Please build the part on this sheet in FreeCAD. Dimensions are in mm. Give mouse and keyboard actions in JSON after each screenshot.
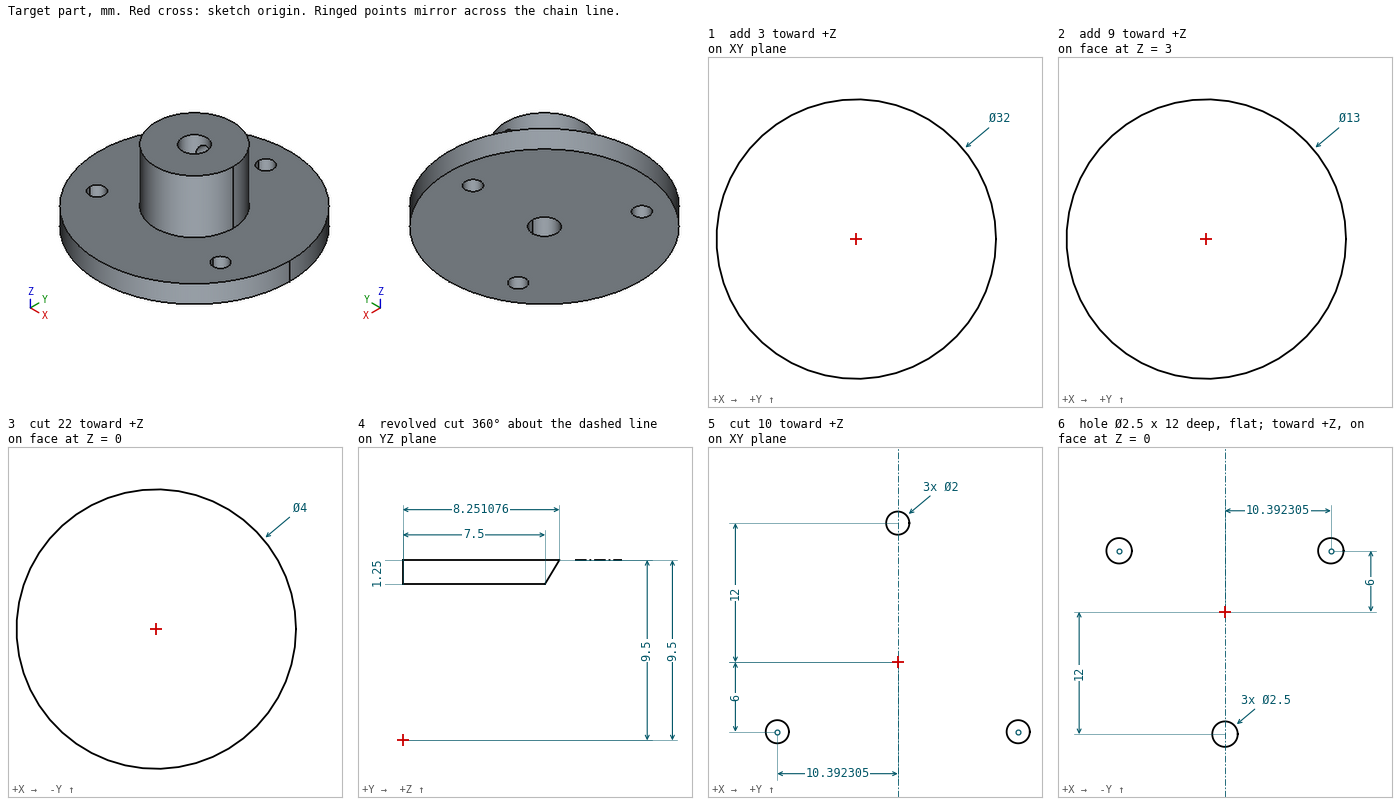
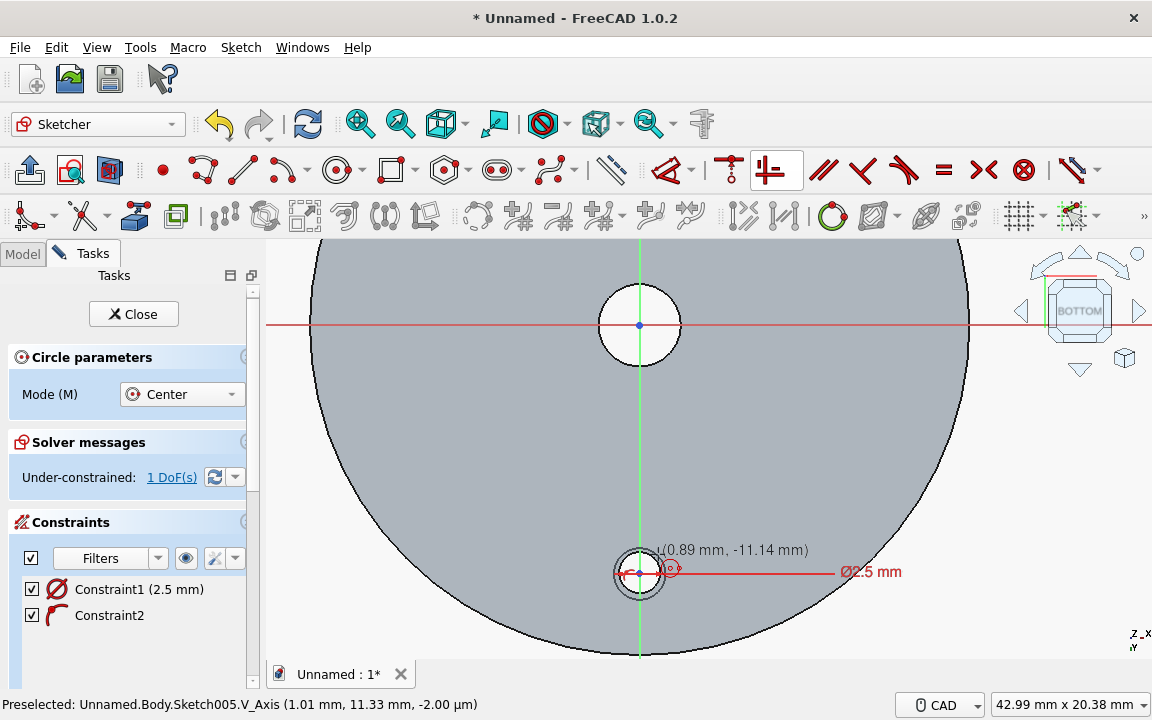
{"action": "scroll", "coordinate": [642, 575], "scroll_direction": "down", "scroll_amount": 2}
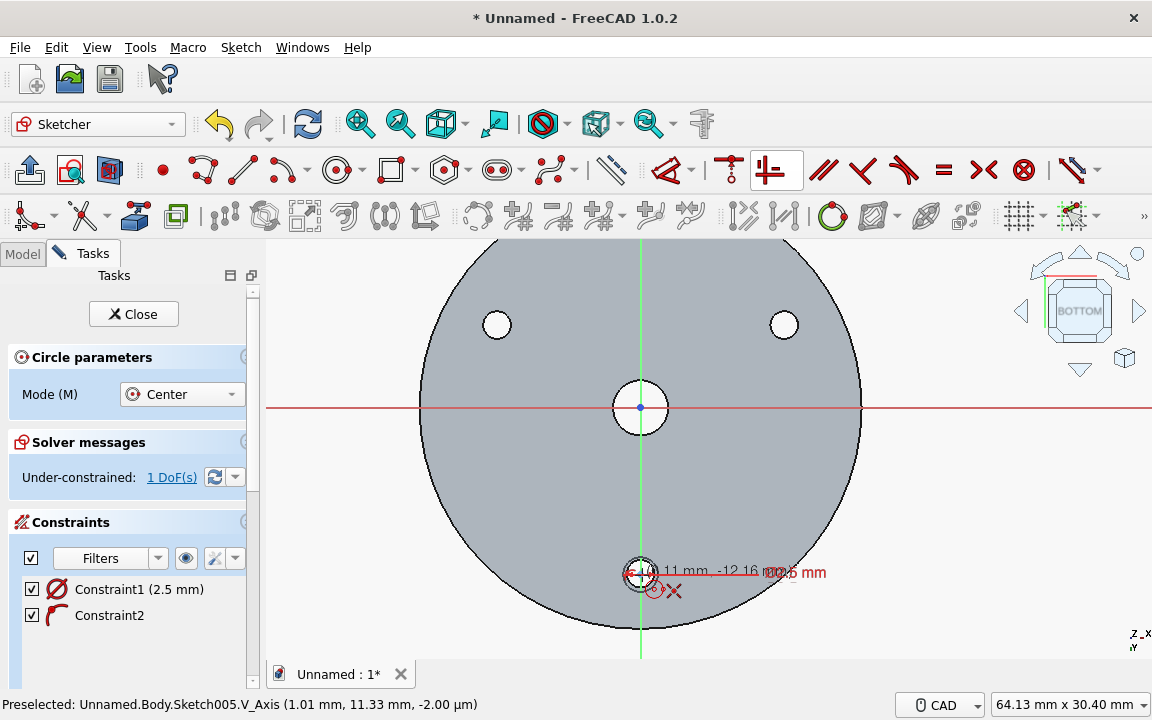
{"action": "scroll", "coordinate": [784, 325], "scroll_direction": "up", "scroll_amount": 2}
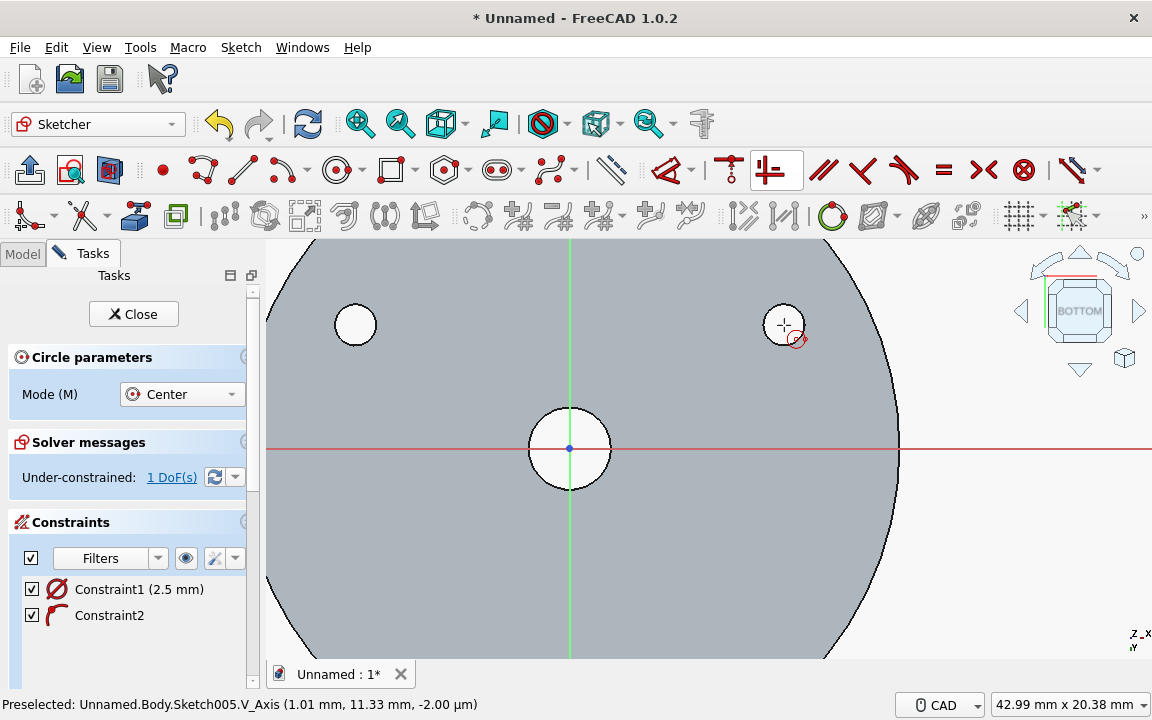
{"action": "left_click", "coordinate": [784, 325]}
{"action": "mouse_move", "coordinate": [802, 307]}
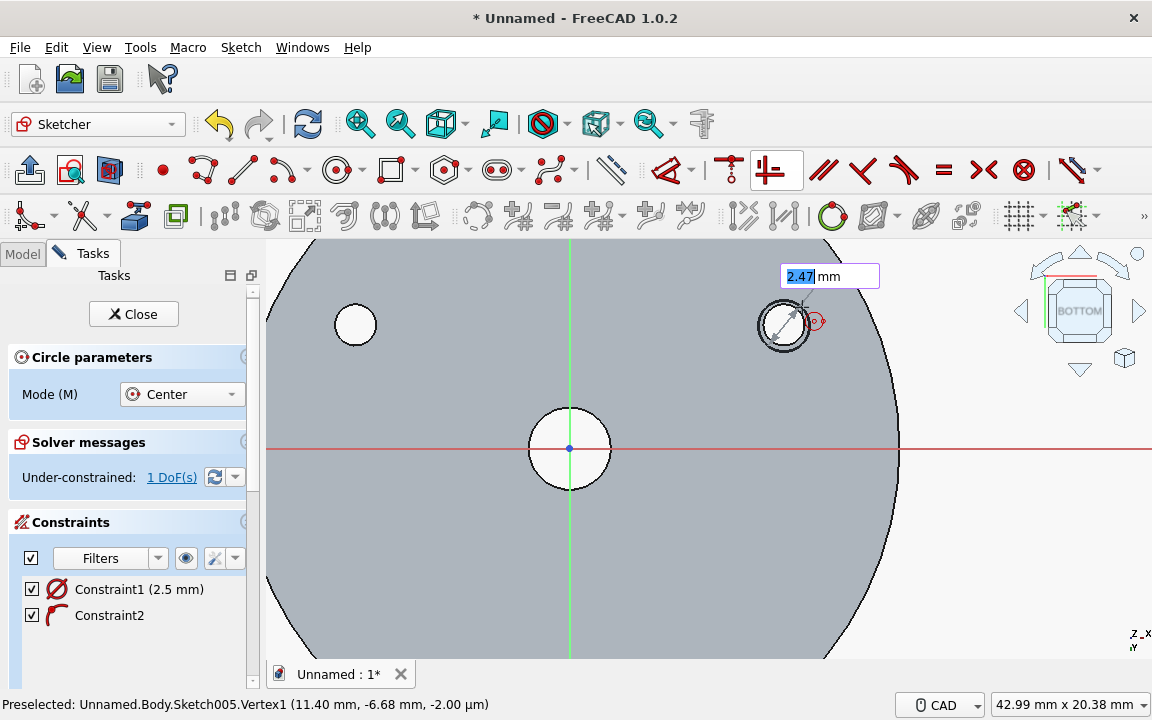
{"action": "type", "text": "2.5"}
{"action": "key", "text": "Return"}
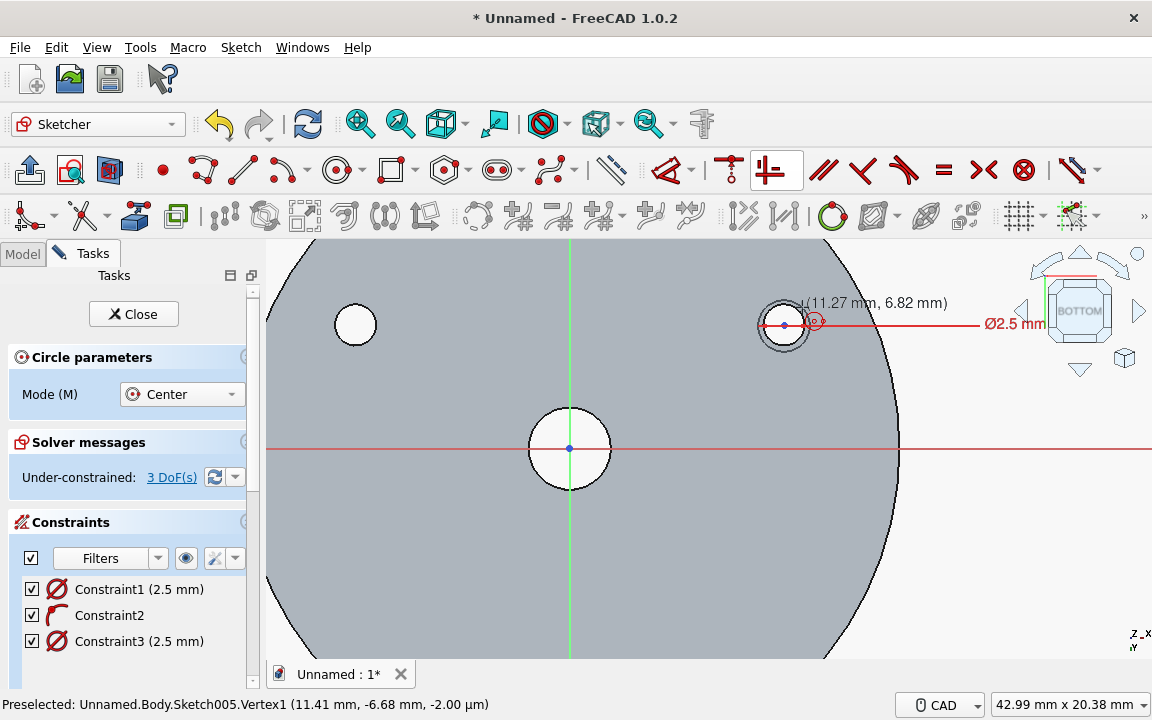
{"action": "left_click", "coordinate": [356, 325]}
{"action": "mouse_move", "coordinate": [374, 307]}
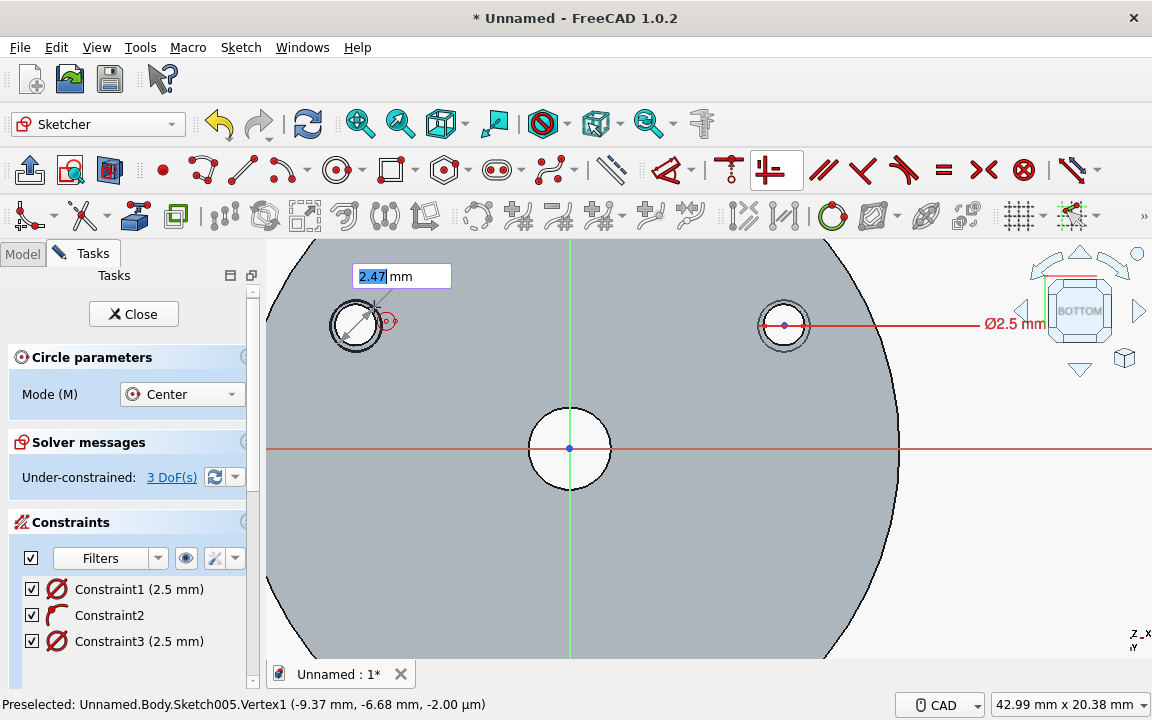
{"action": "type", "text": "2.5"}
{"action": "key", "text": "Return"}
{"action": "key", "text": "Escape"}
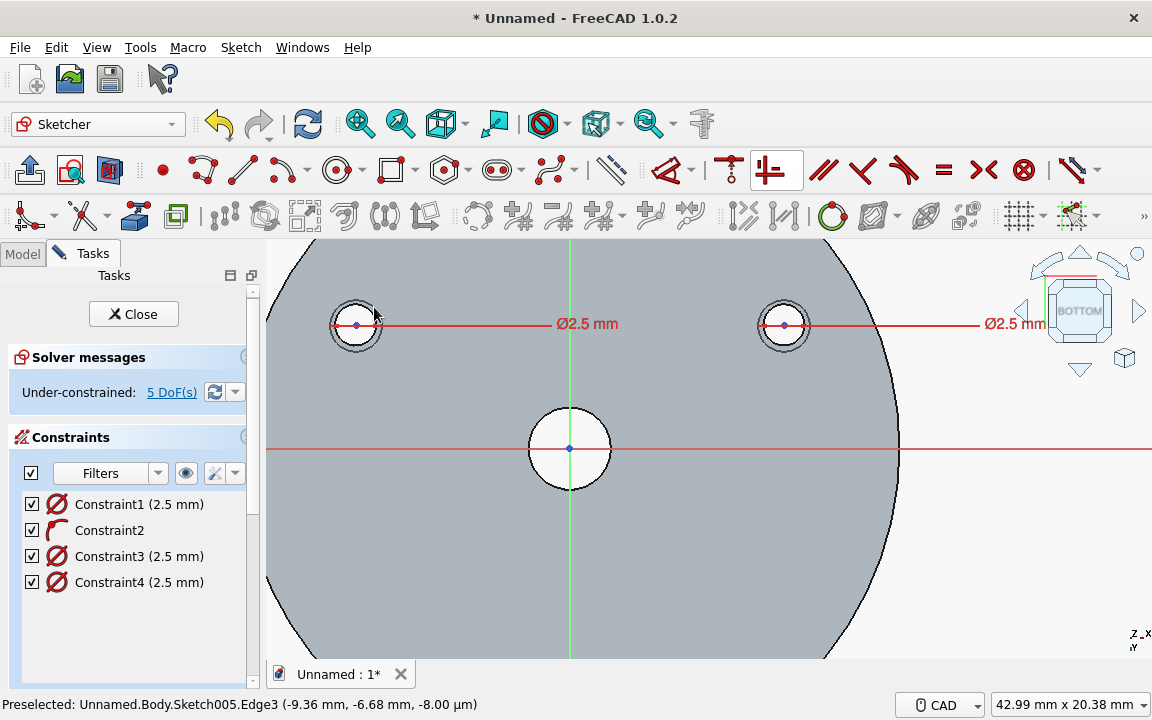
{"action": "left_click", "coordinate": [784, 326]}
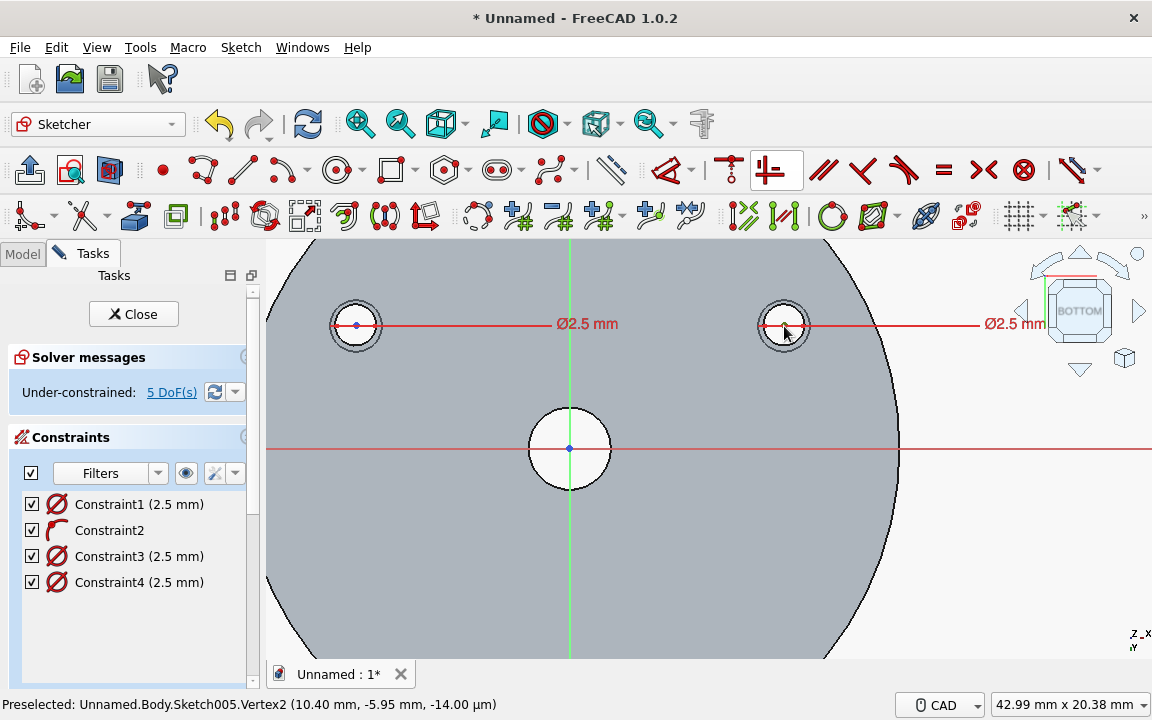
{"action": "left_click", "coordinate": [356, 326]}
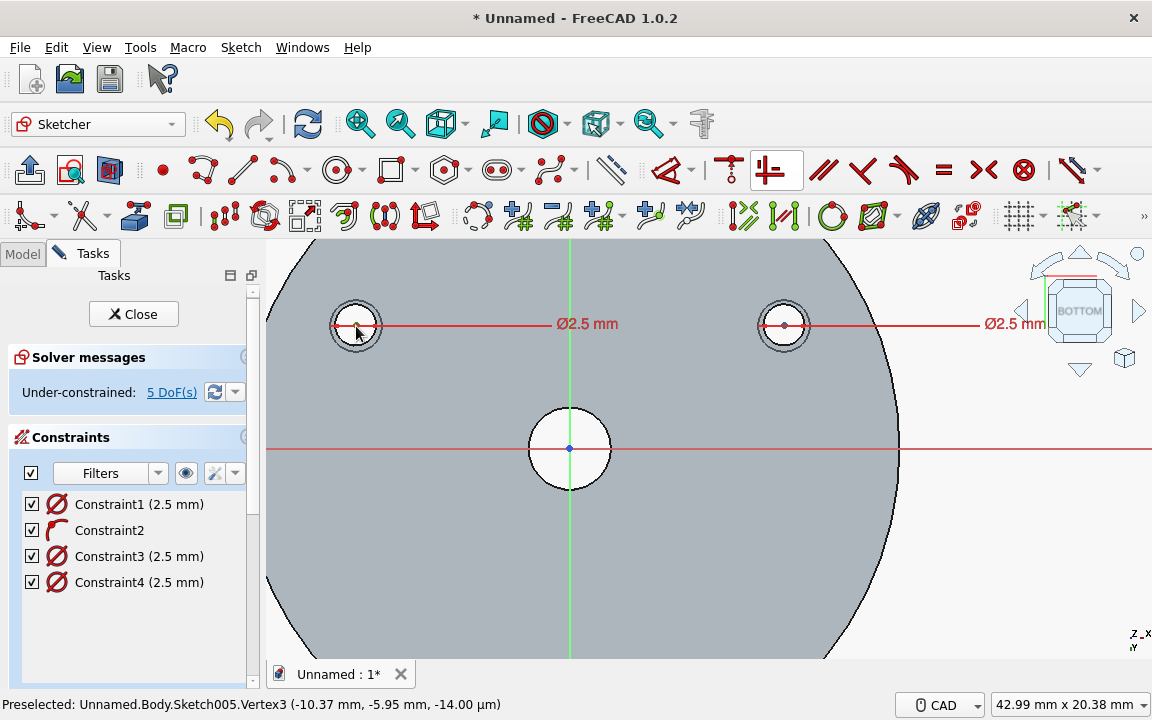
{"action": "left_click", "coordinate": [570, 605]}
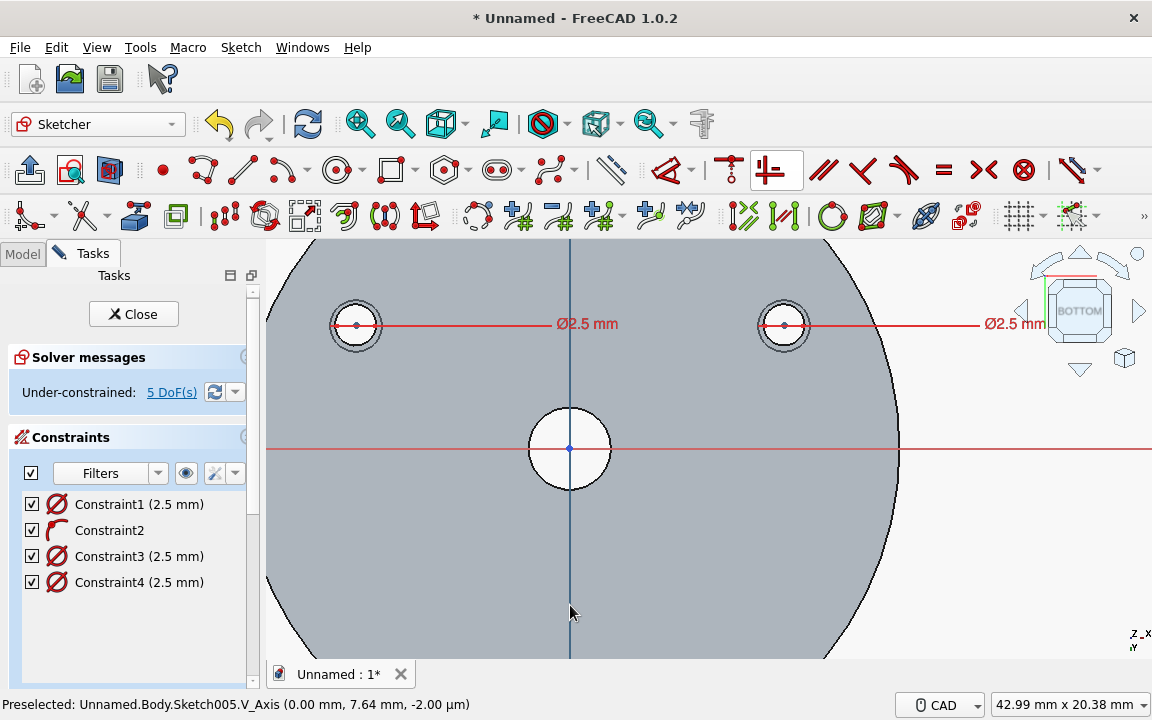
{"action": "left_click", "coordinate": [984, 170]}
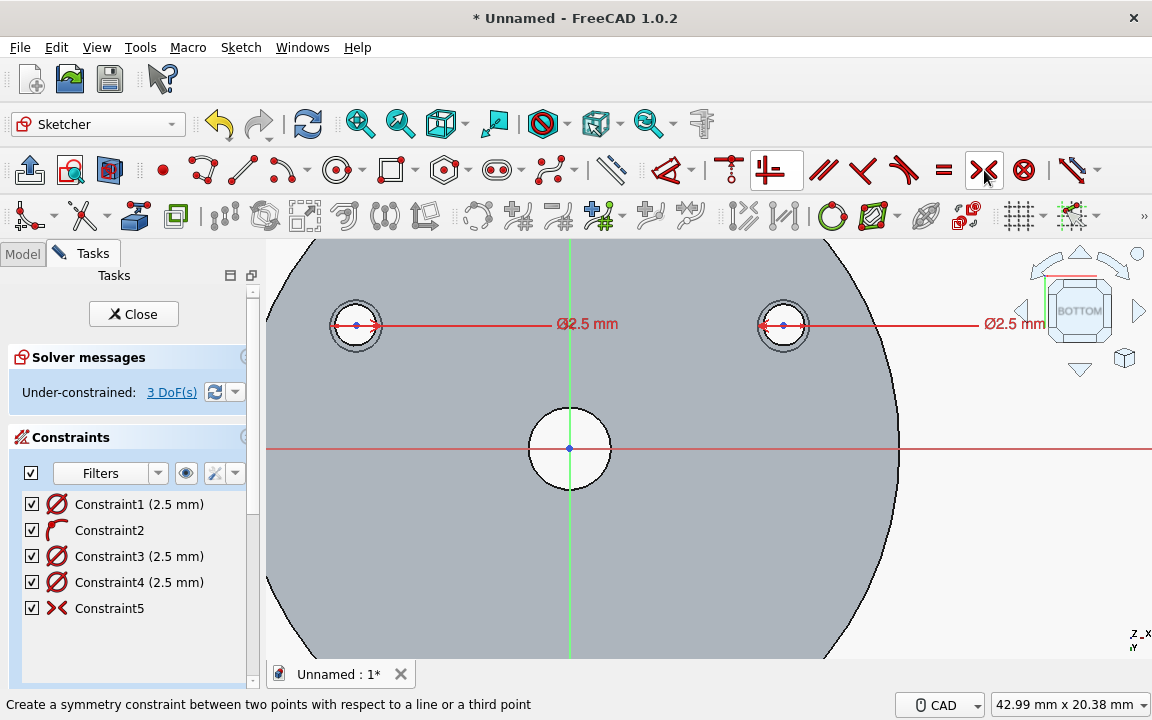
{"action": "left_click", "coordinate": [666, 170]}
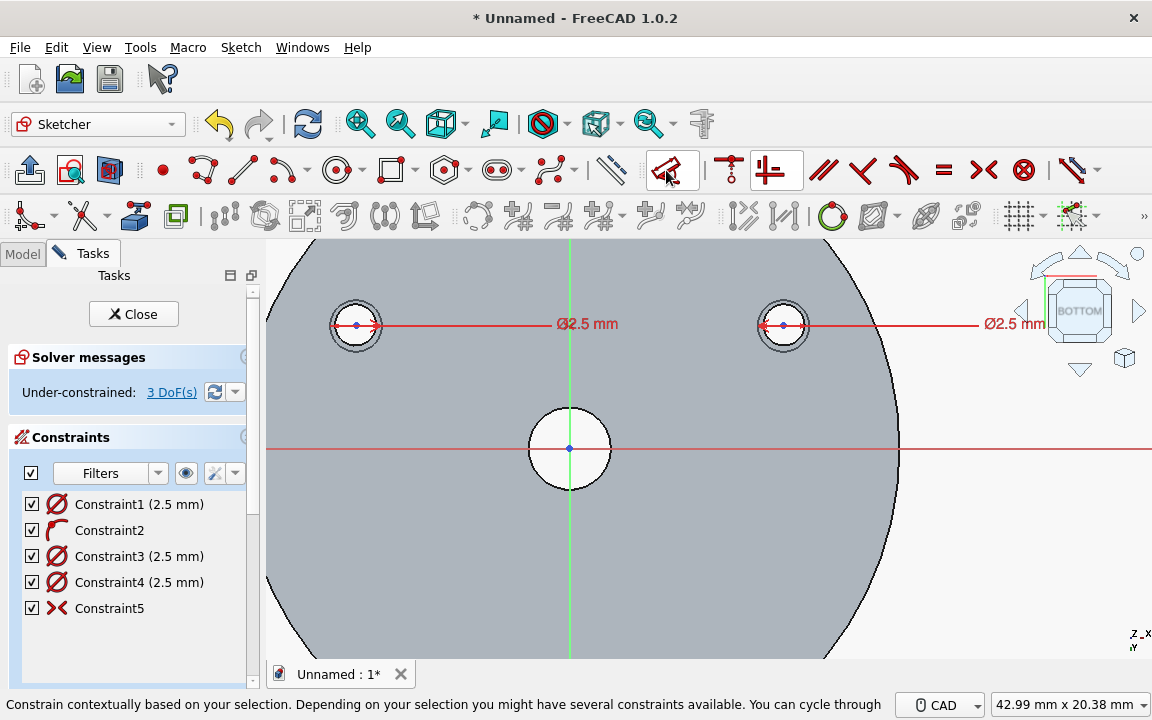
{"action": "left_click", "coordinate": [784, 326]}
{"action": "left_click", "coordinate": [818, 387]}